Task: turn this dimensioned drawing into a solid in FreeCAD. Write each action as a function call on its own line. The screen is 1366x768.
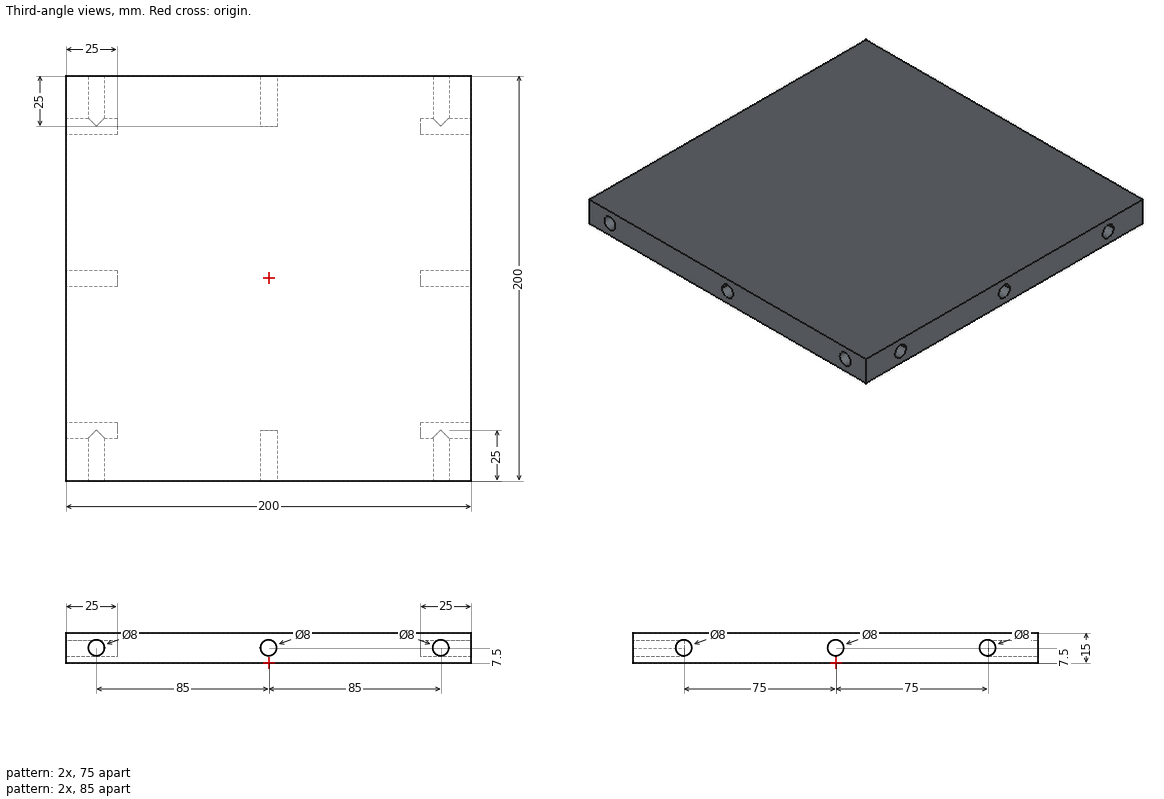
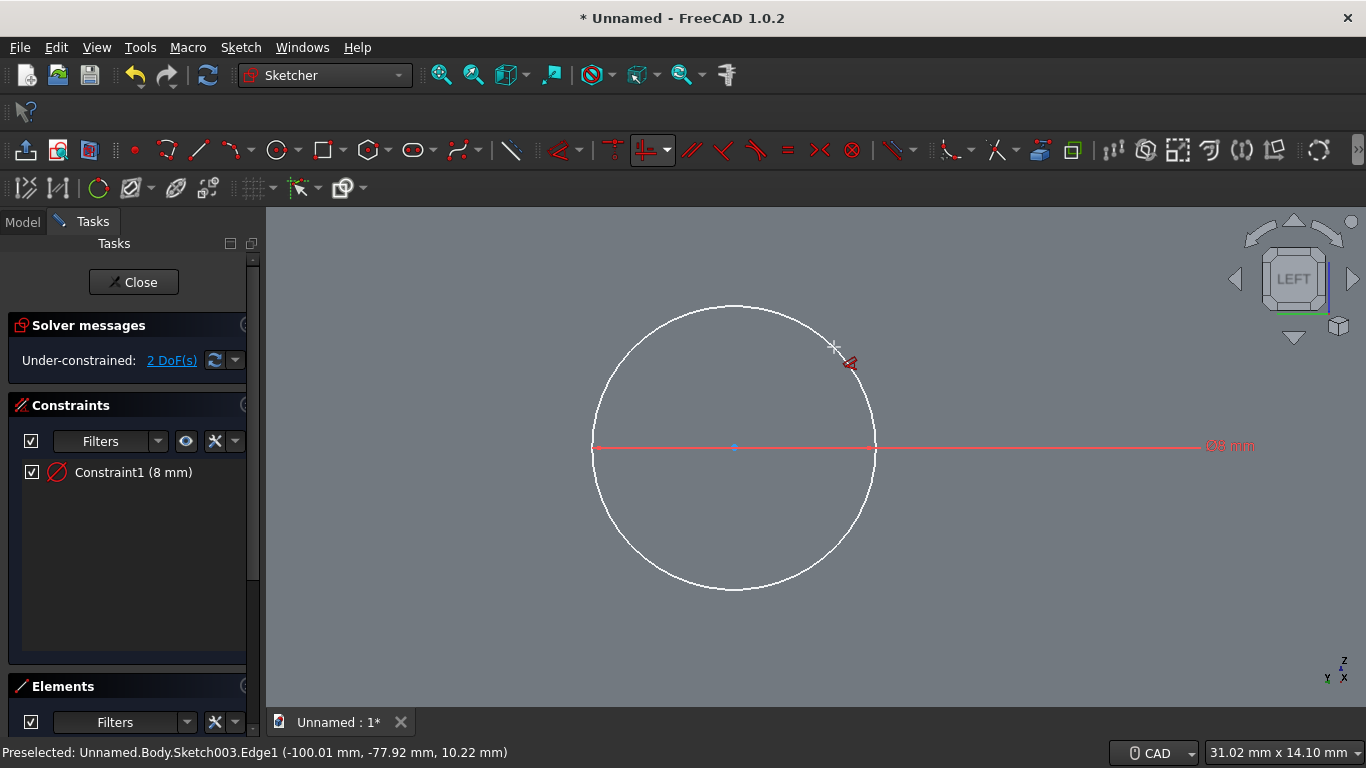
click(734, 448)
click(514, 414)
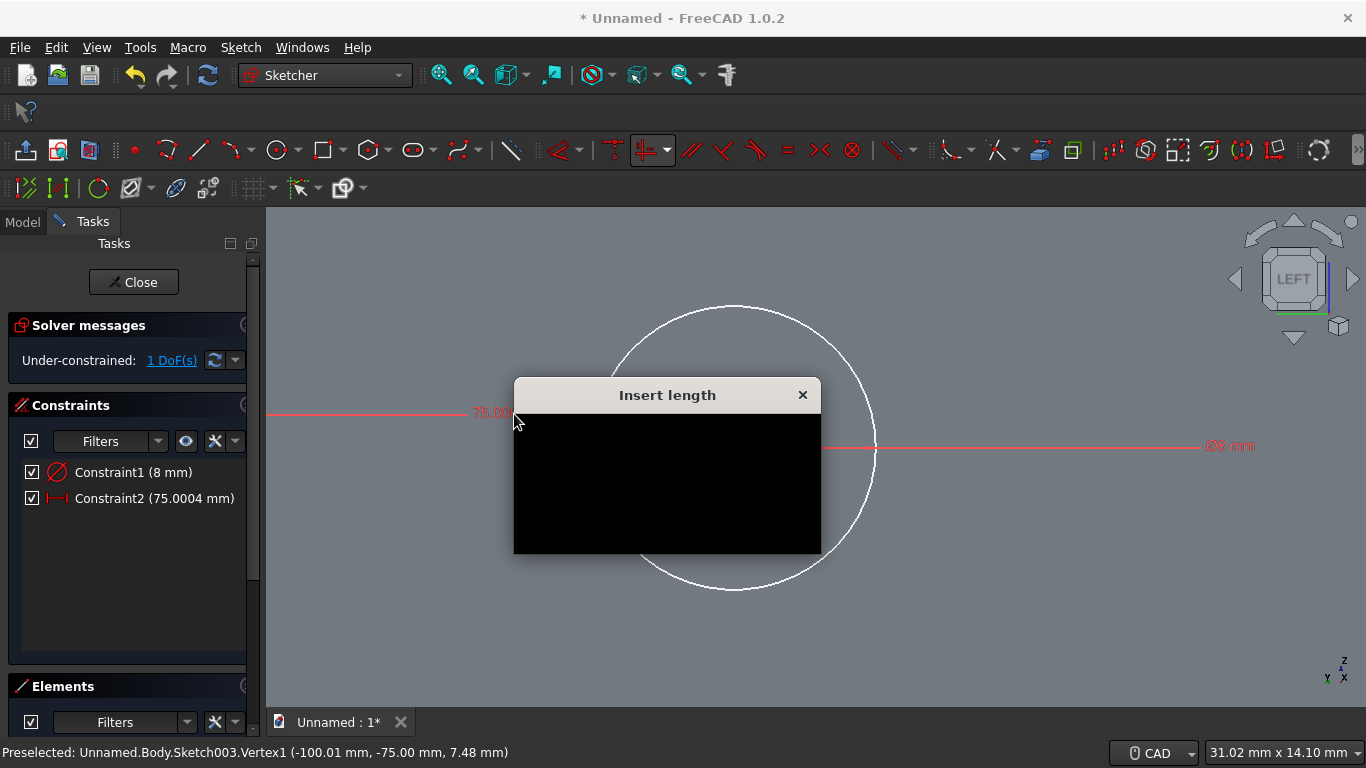
text(75)
key(Return)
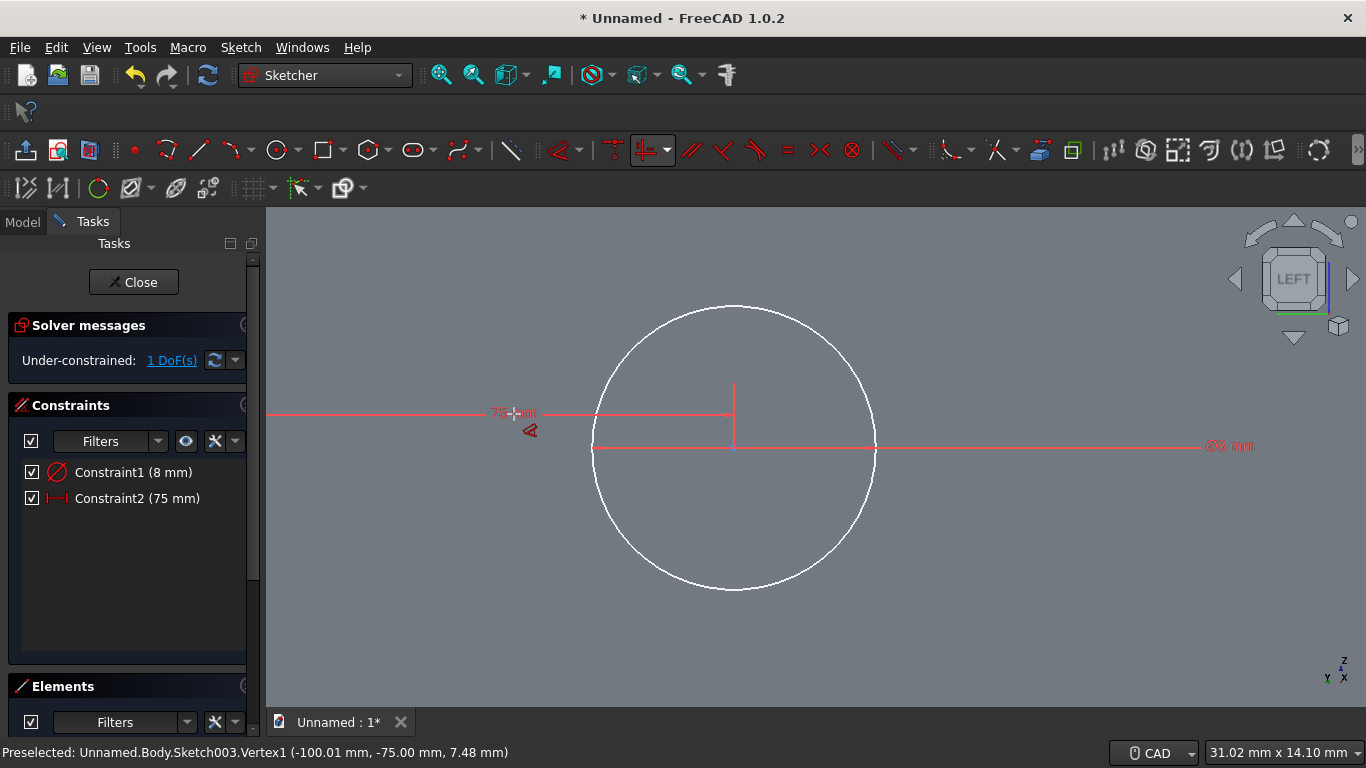
click(734, 448)
click(768, 564)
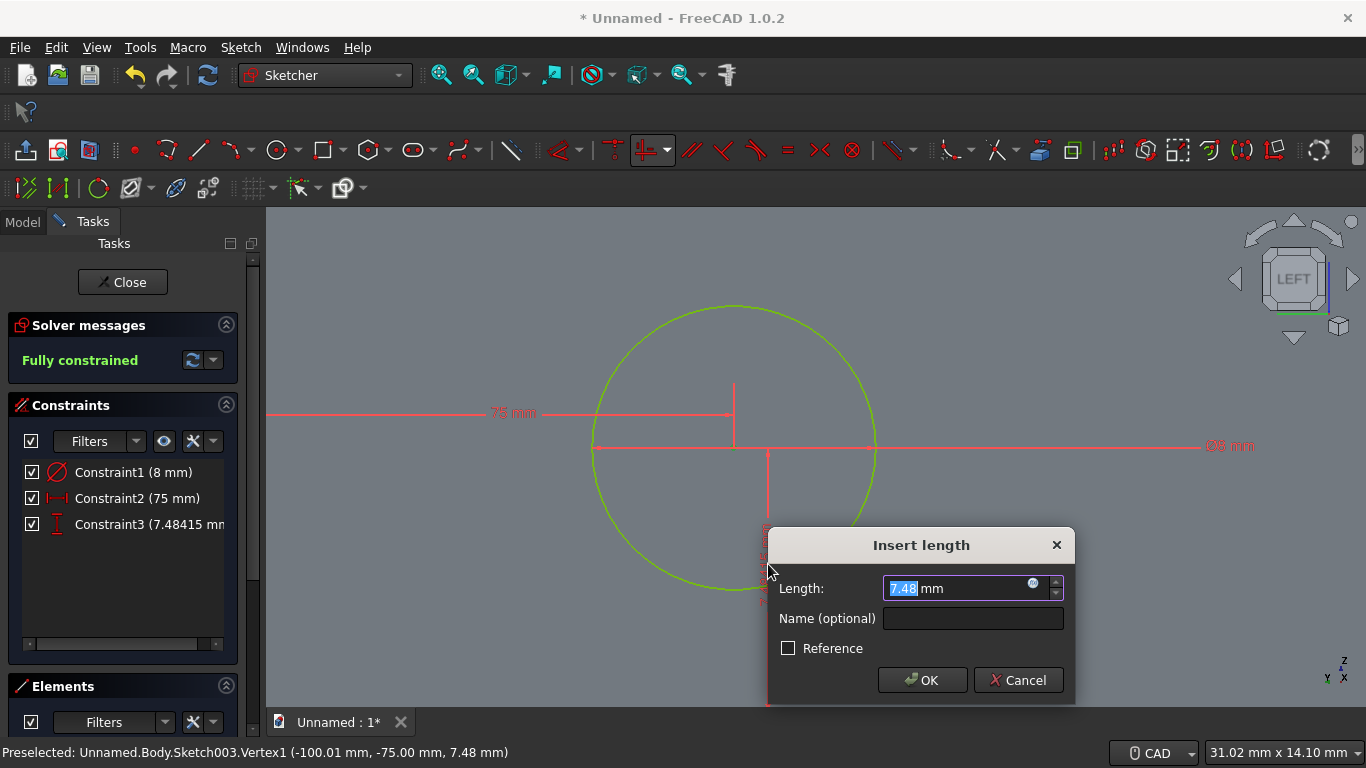
text(7.5)
key(Return)
key(Escape)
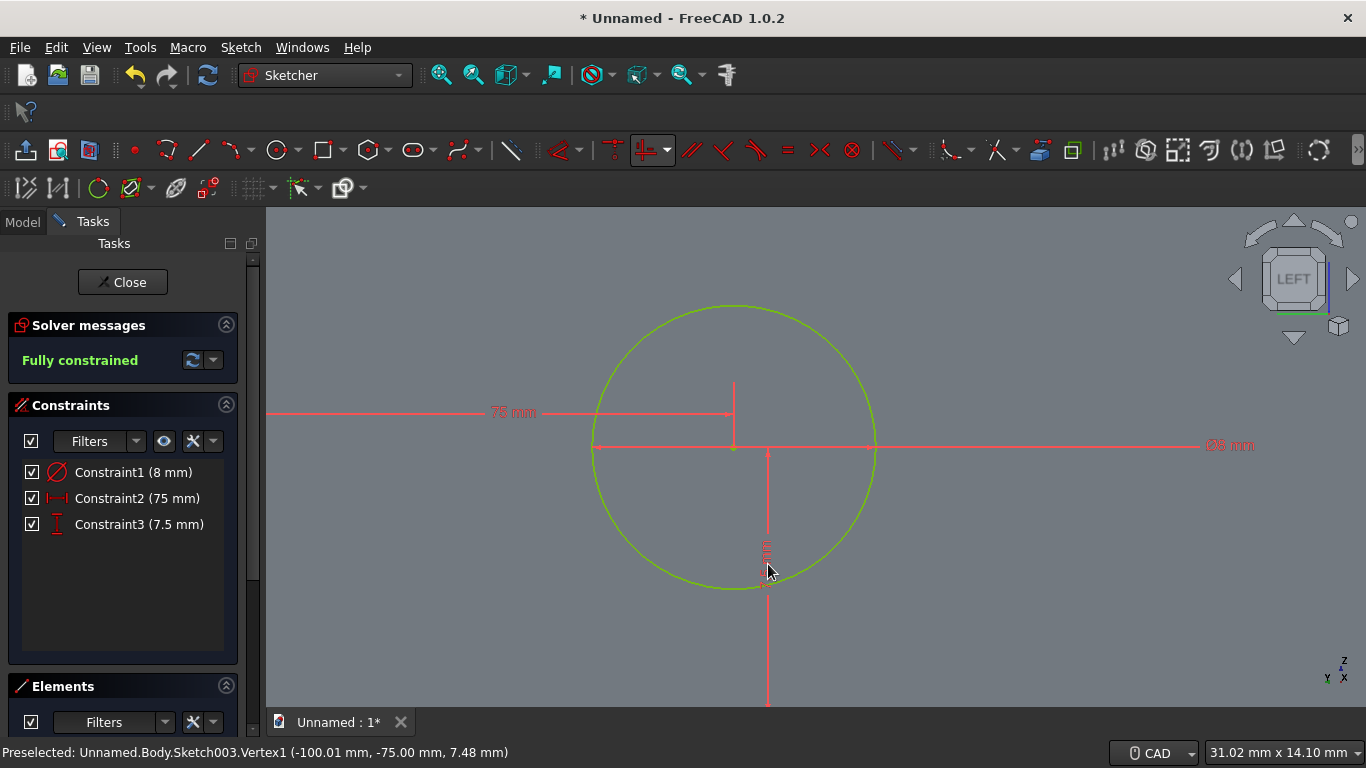
click(123, 282)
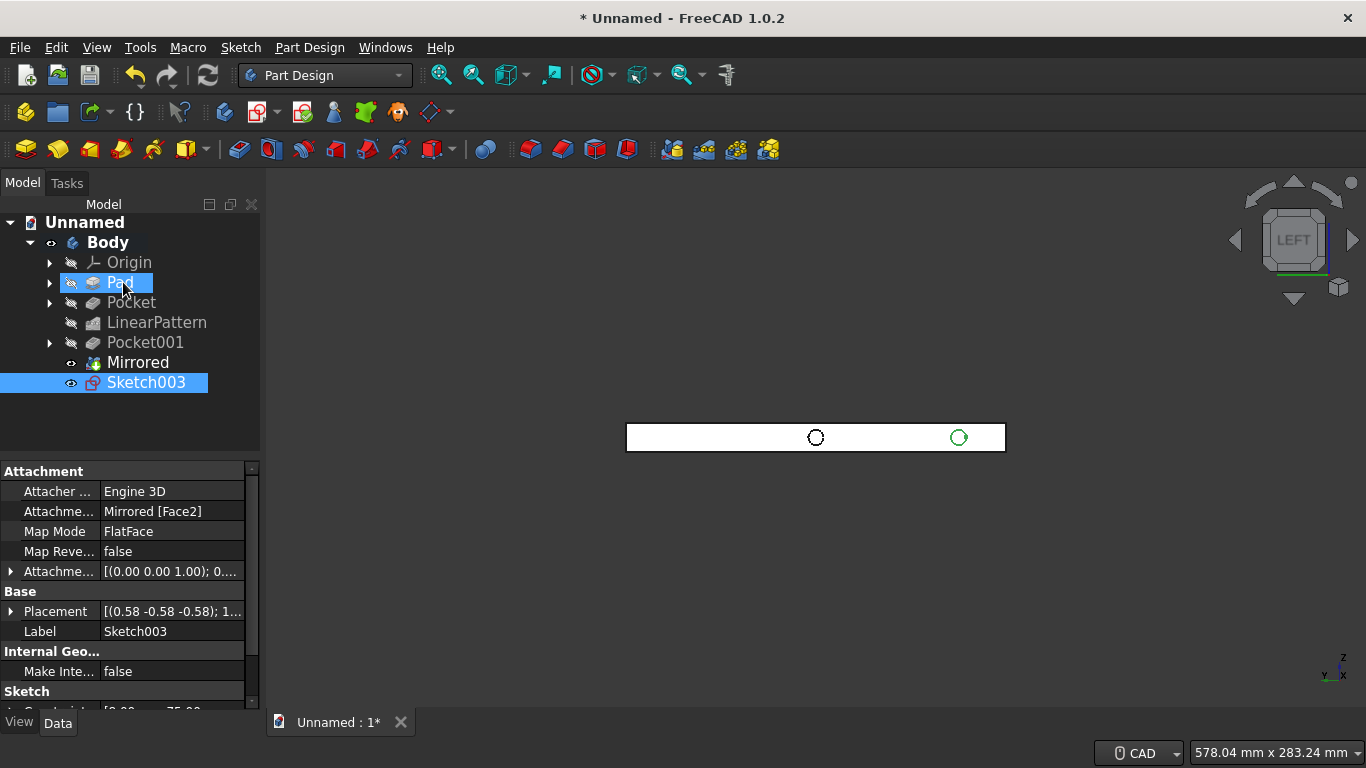
click(240, 150)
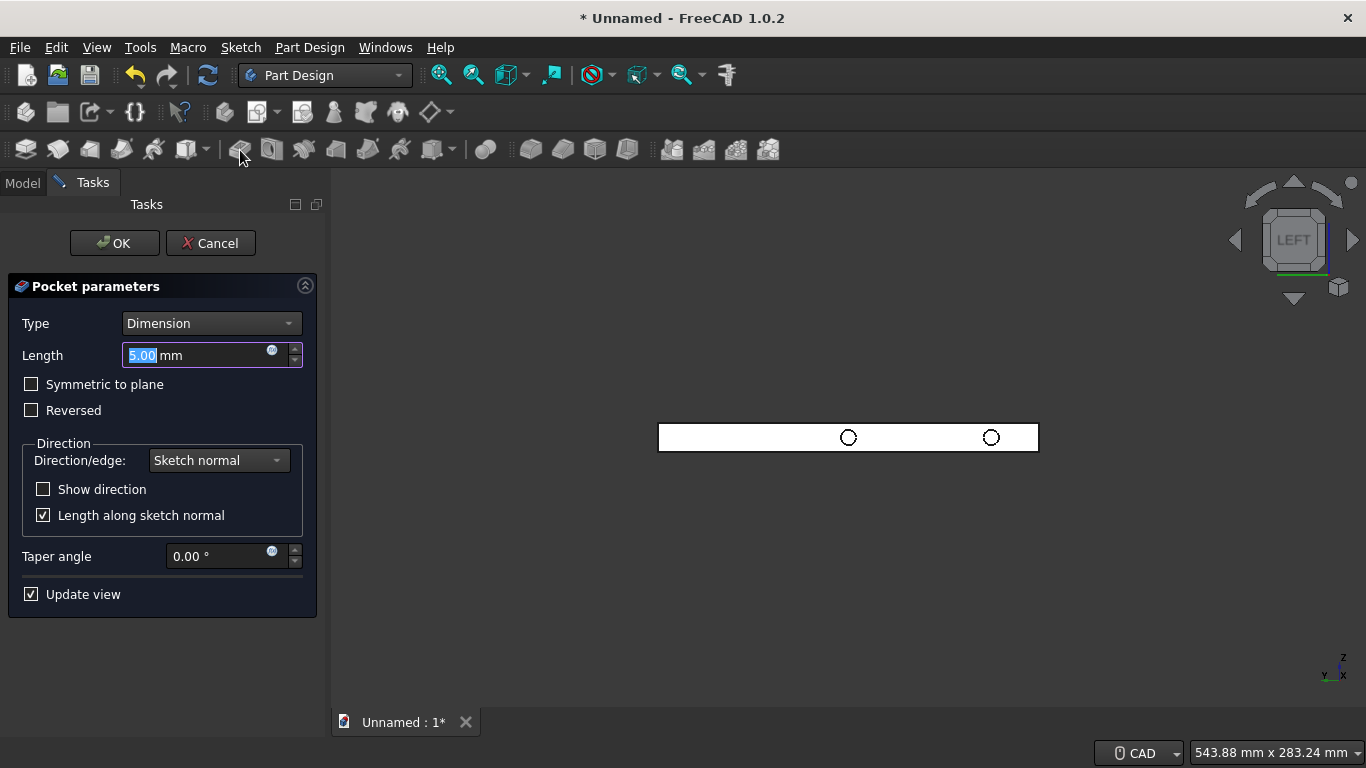
text(25)
key(Tab)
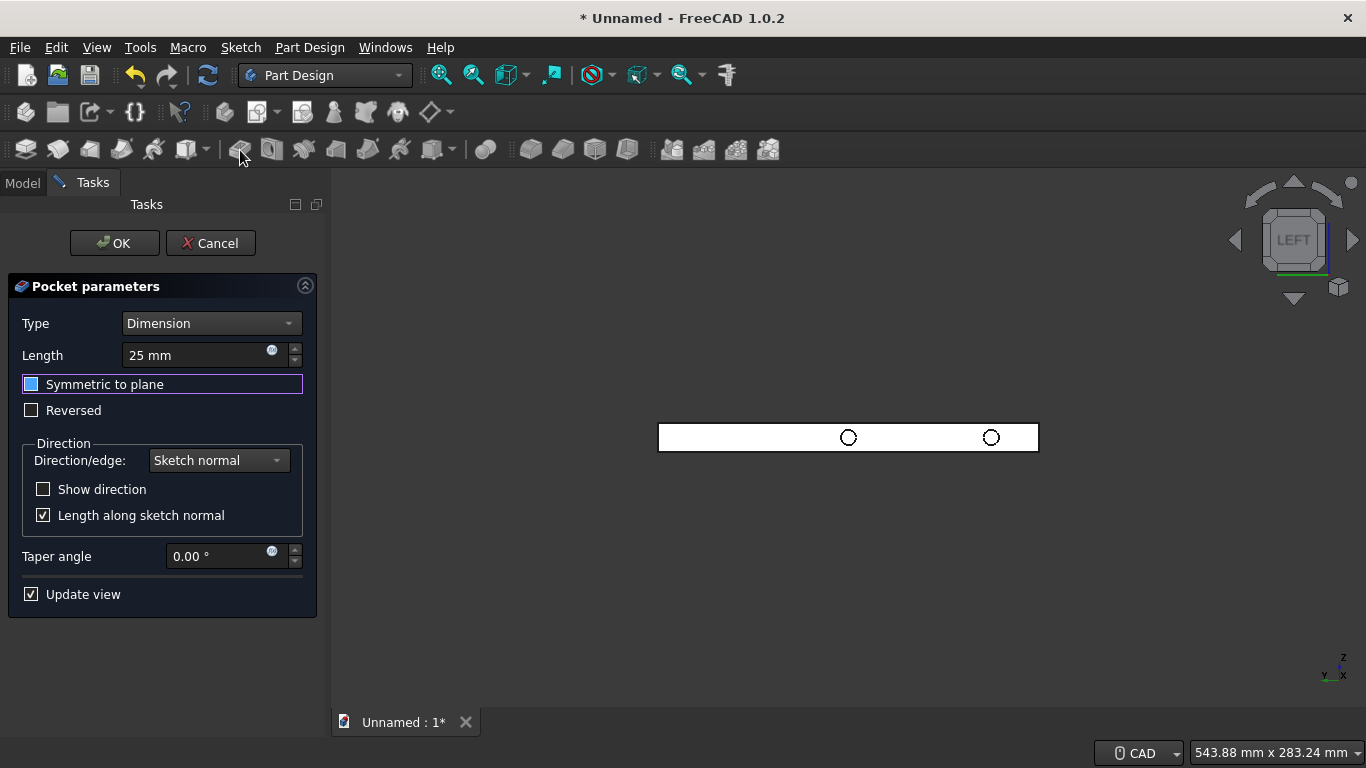
click(115, 243)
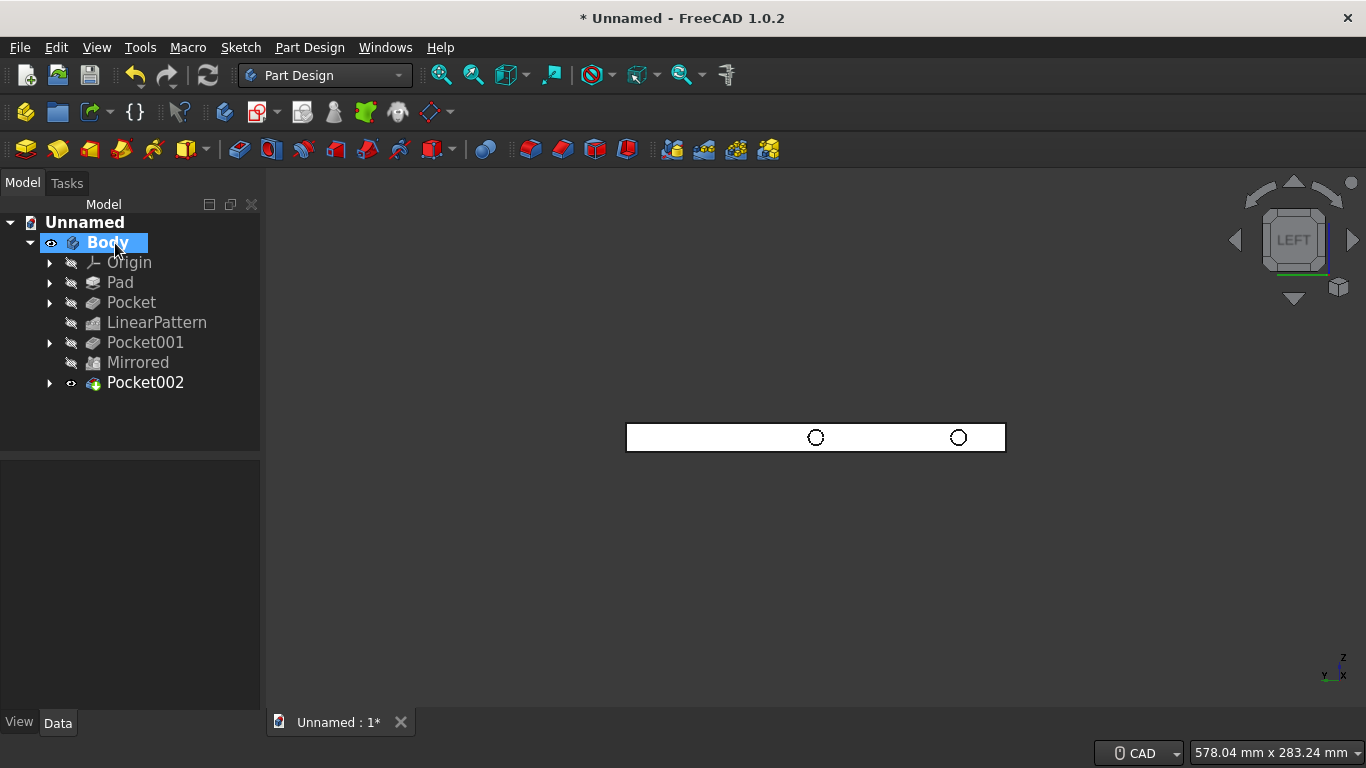
key(v)
key(f)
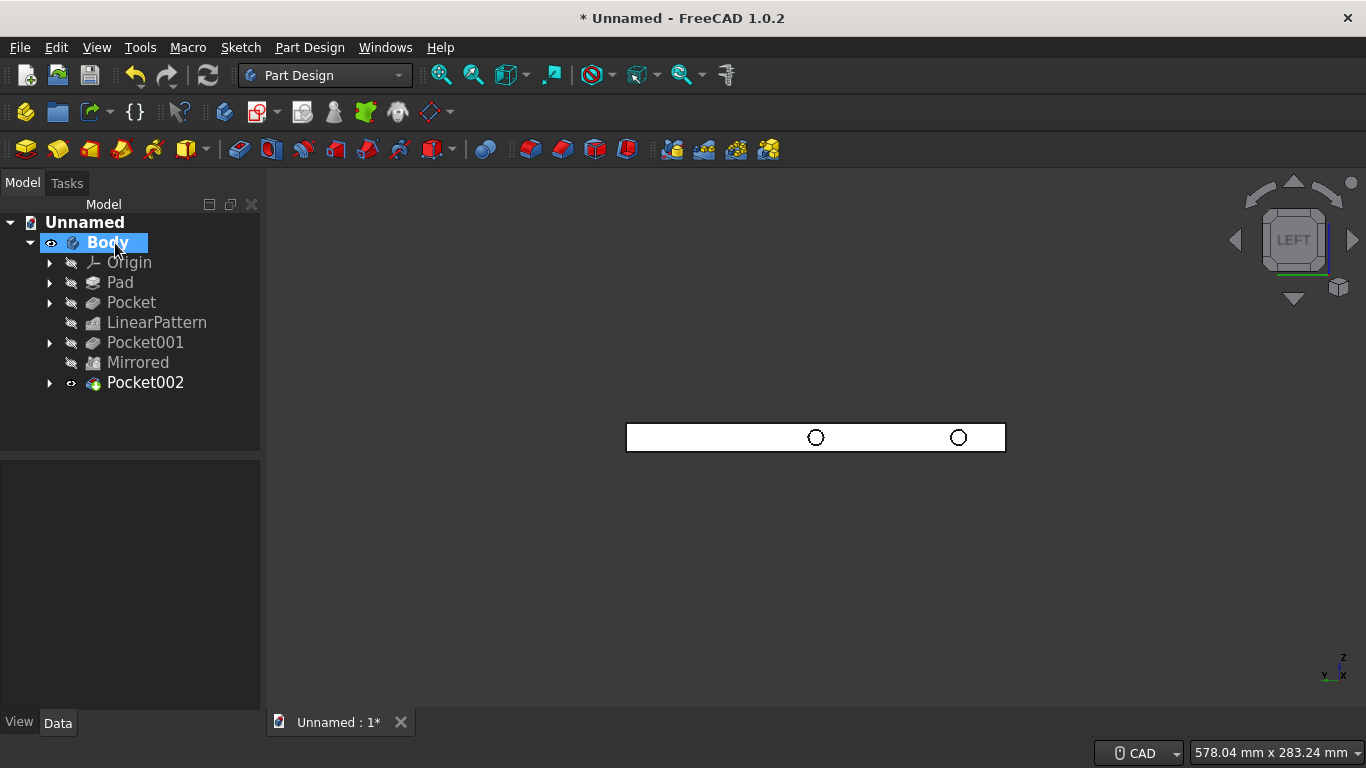
click(653, 436)